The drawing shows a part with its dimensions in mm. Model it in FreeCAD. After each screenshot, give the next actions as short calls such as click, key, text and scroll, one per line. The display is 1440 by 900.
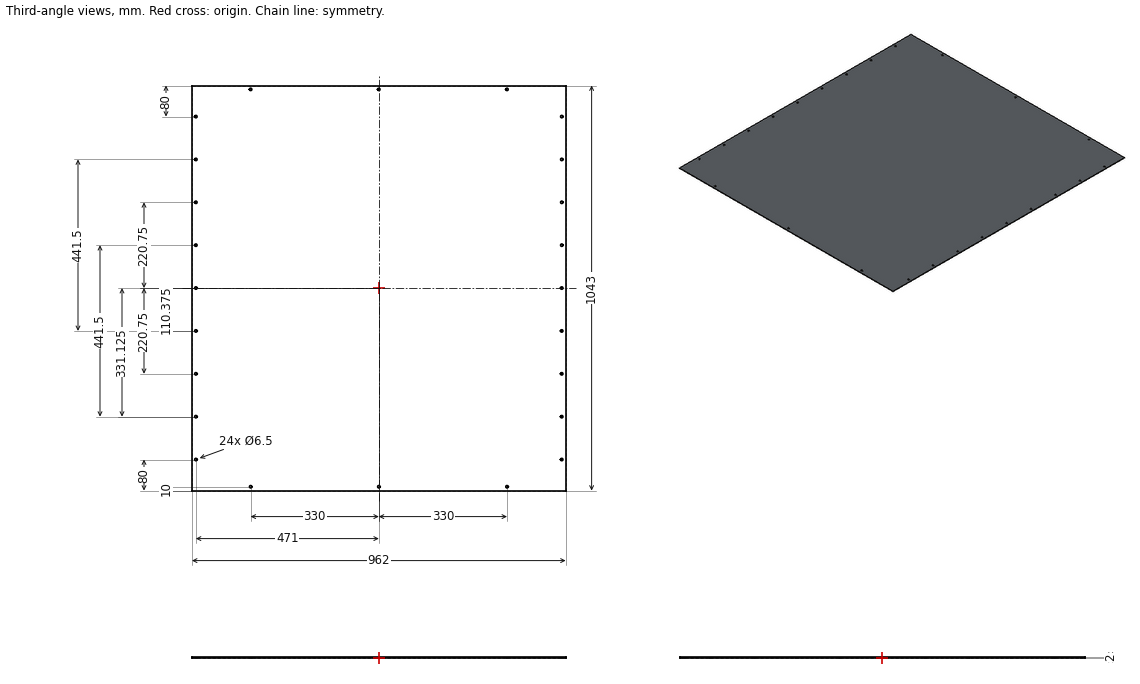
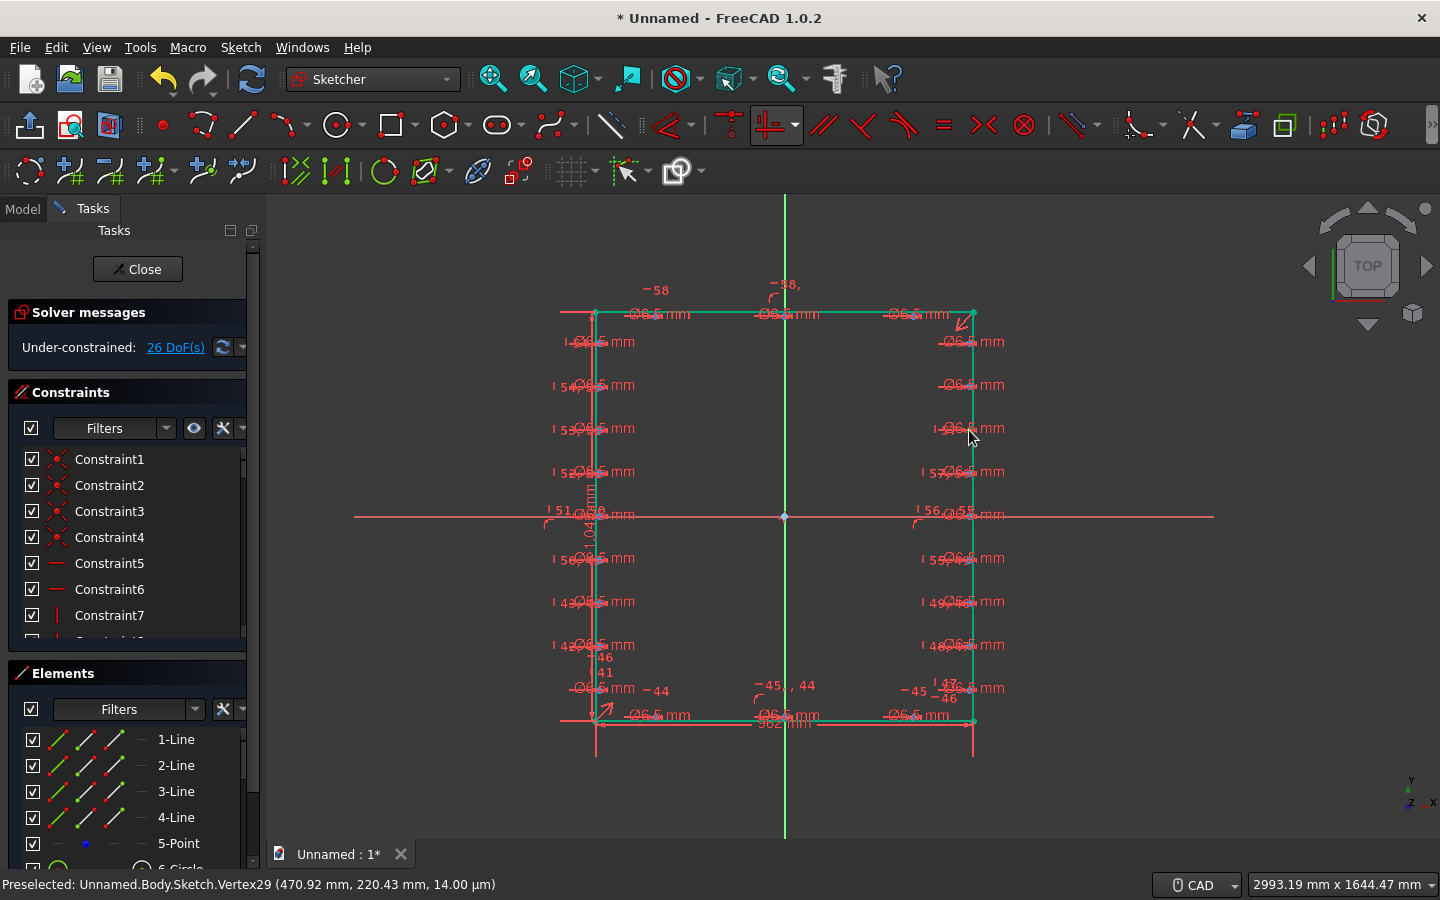
click(969, 387)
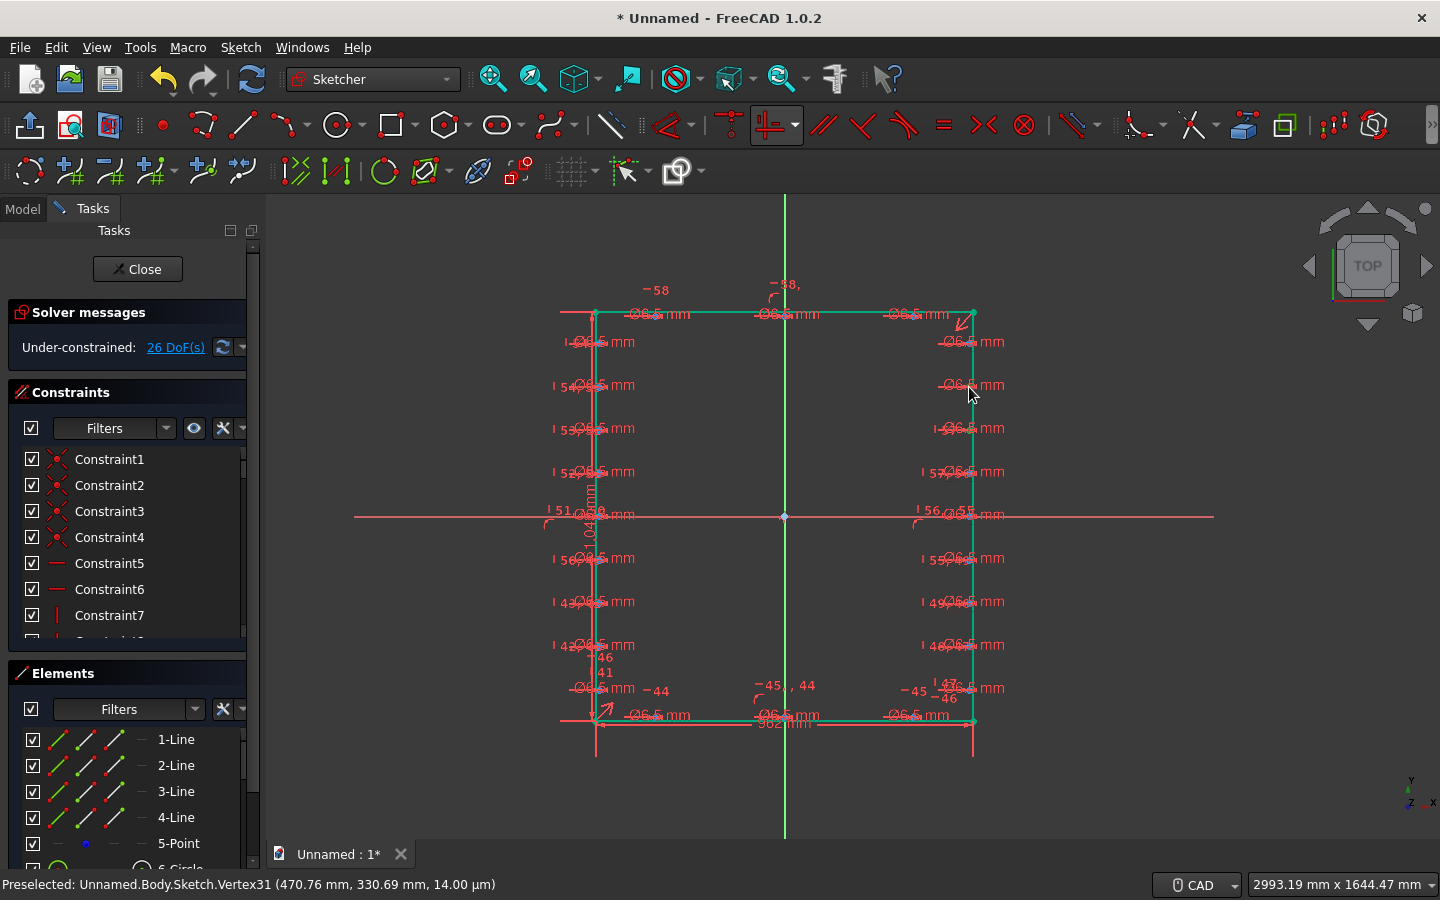
click(798, 126)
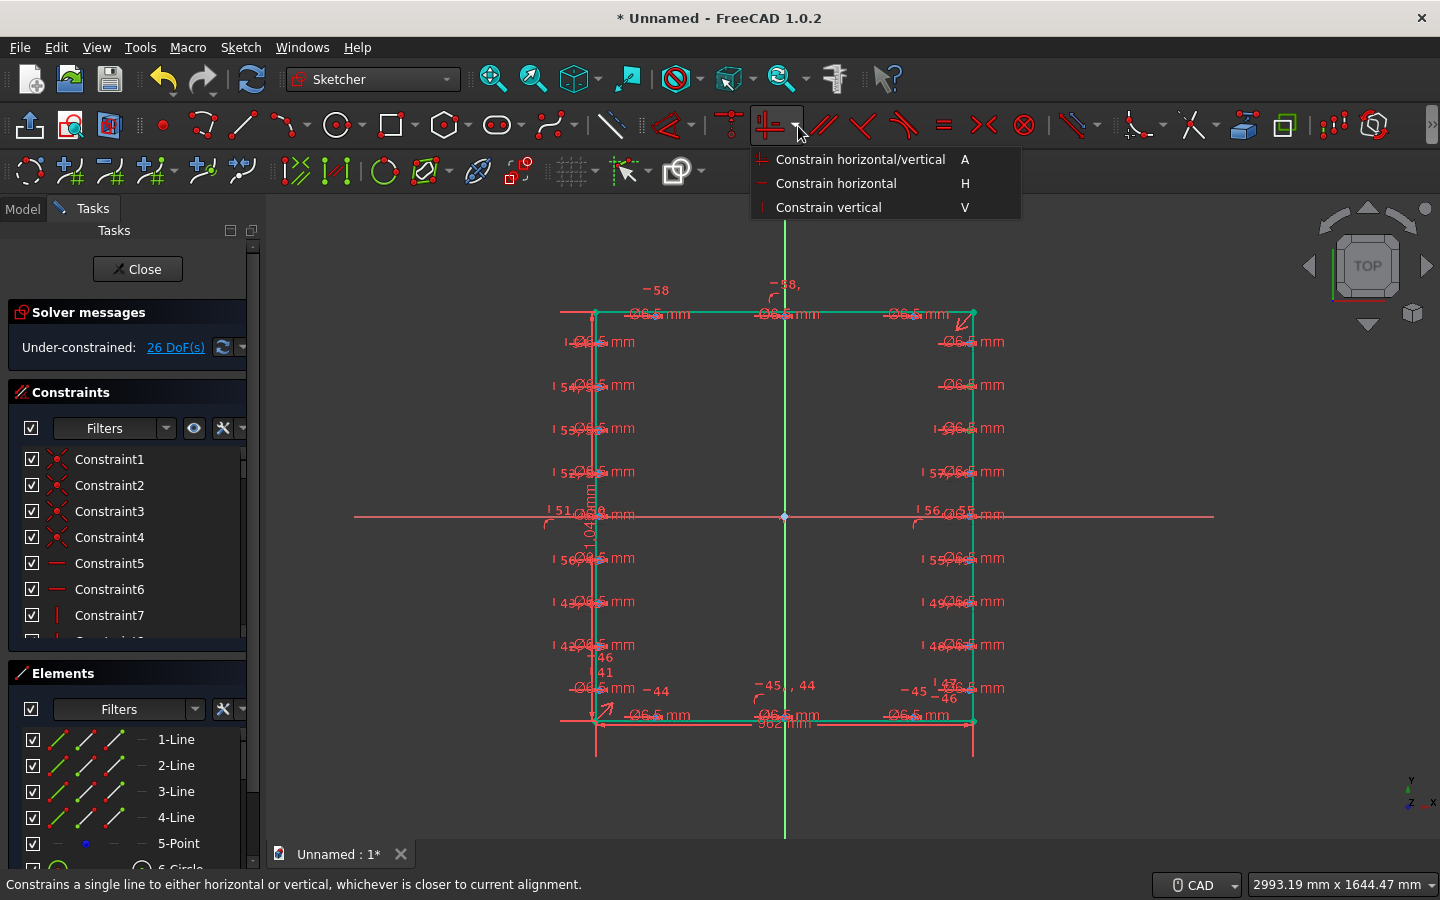
click(886, 207)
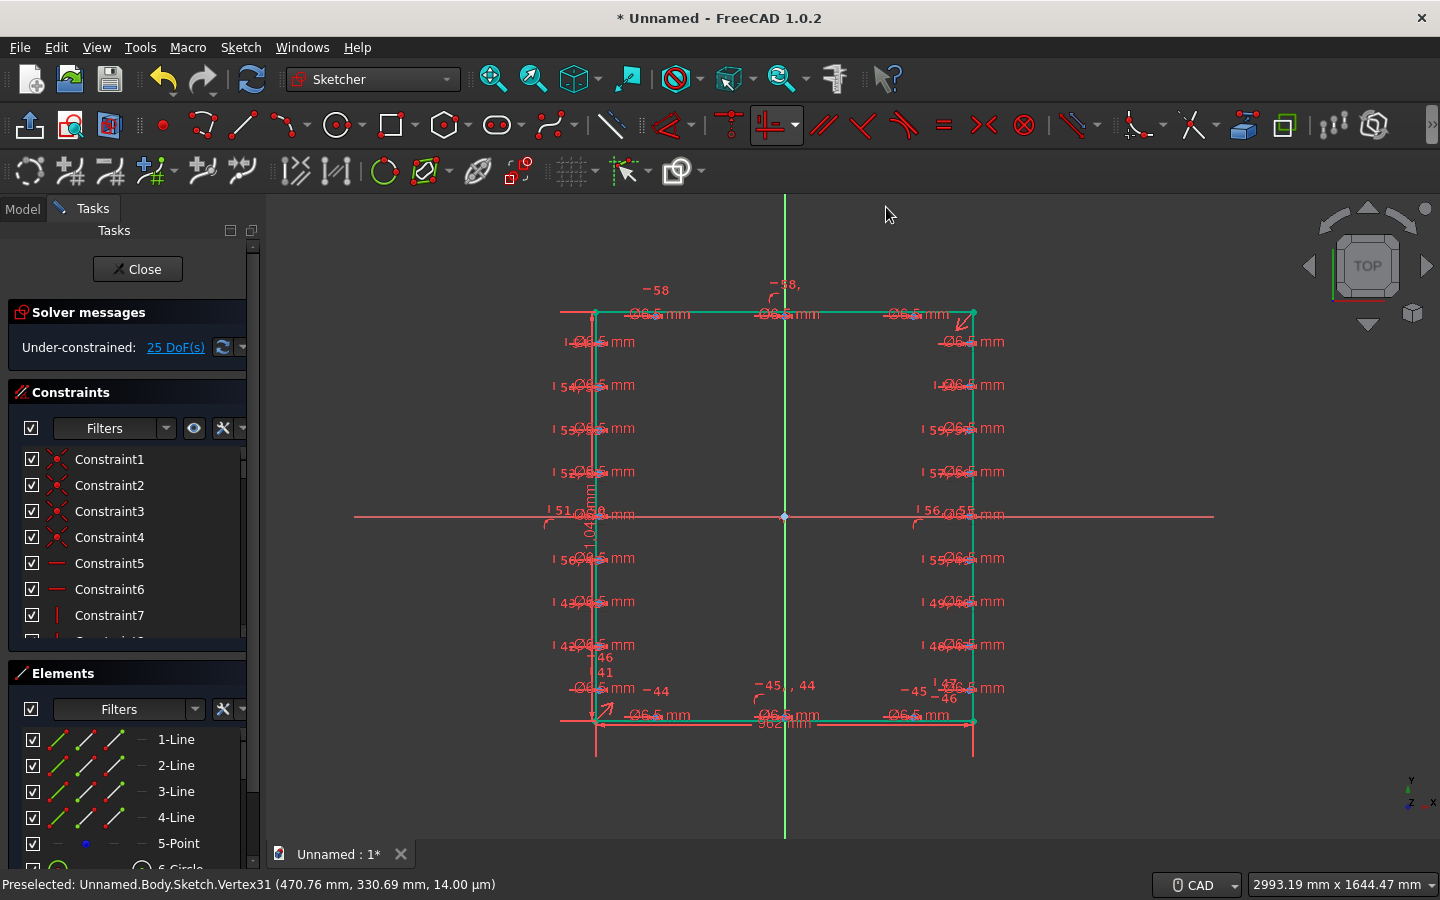
click(785, 316)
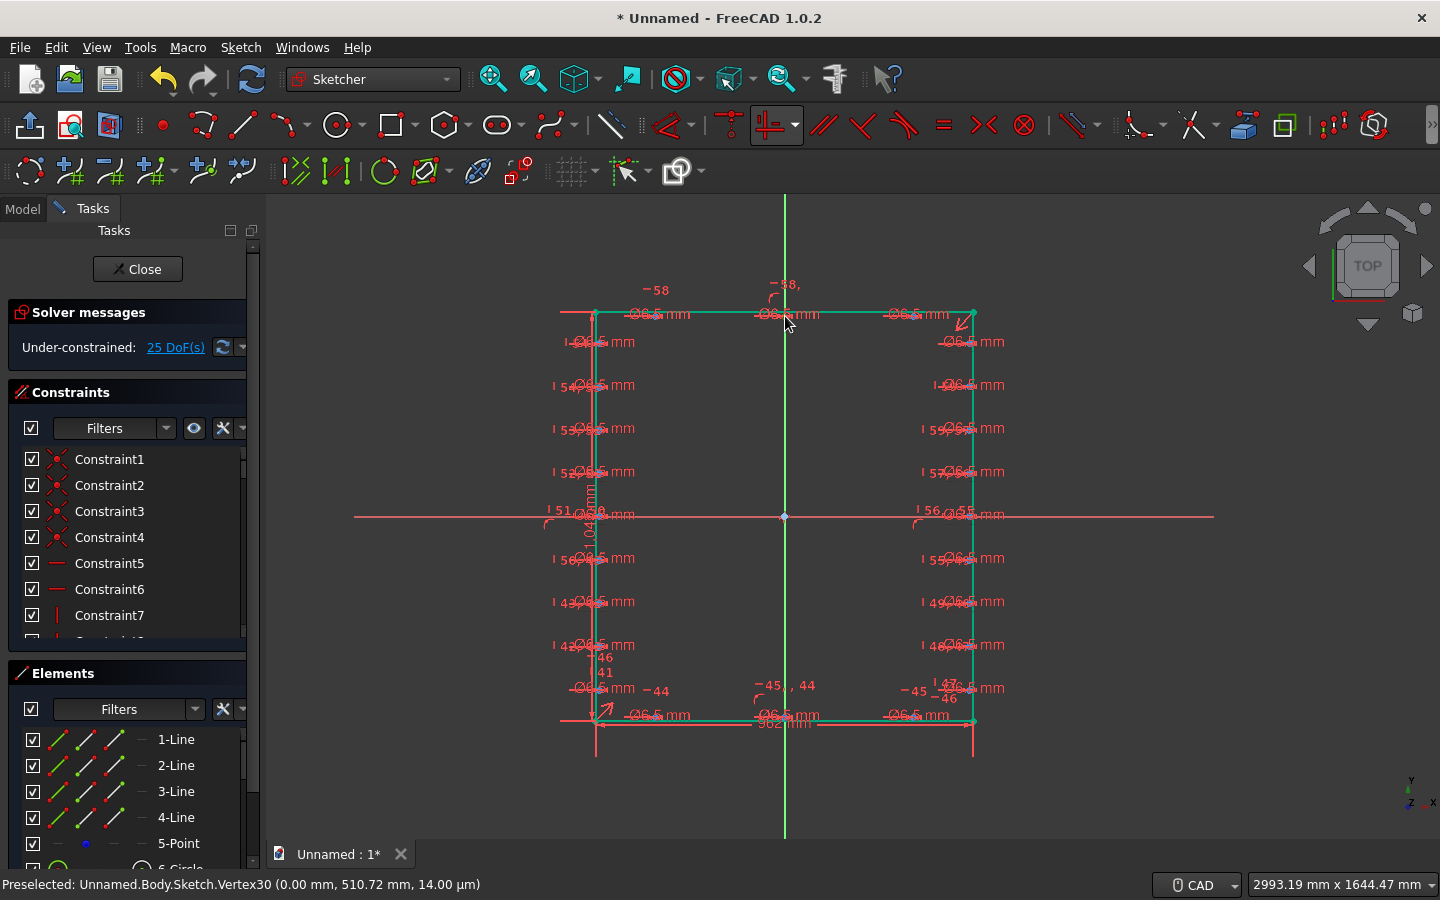
click(914, 316)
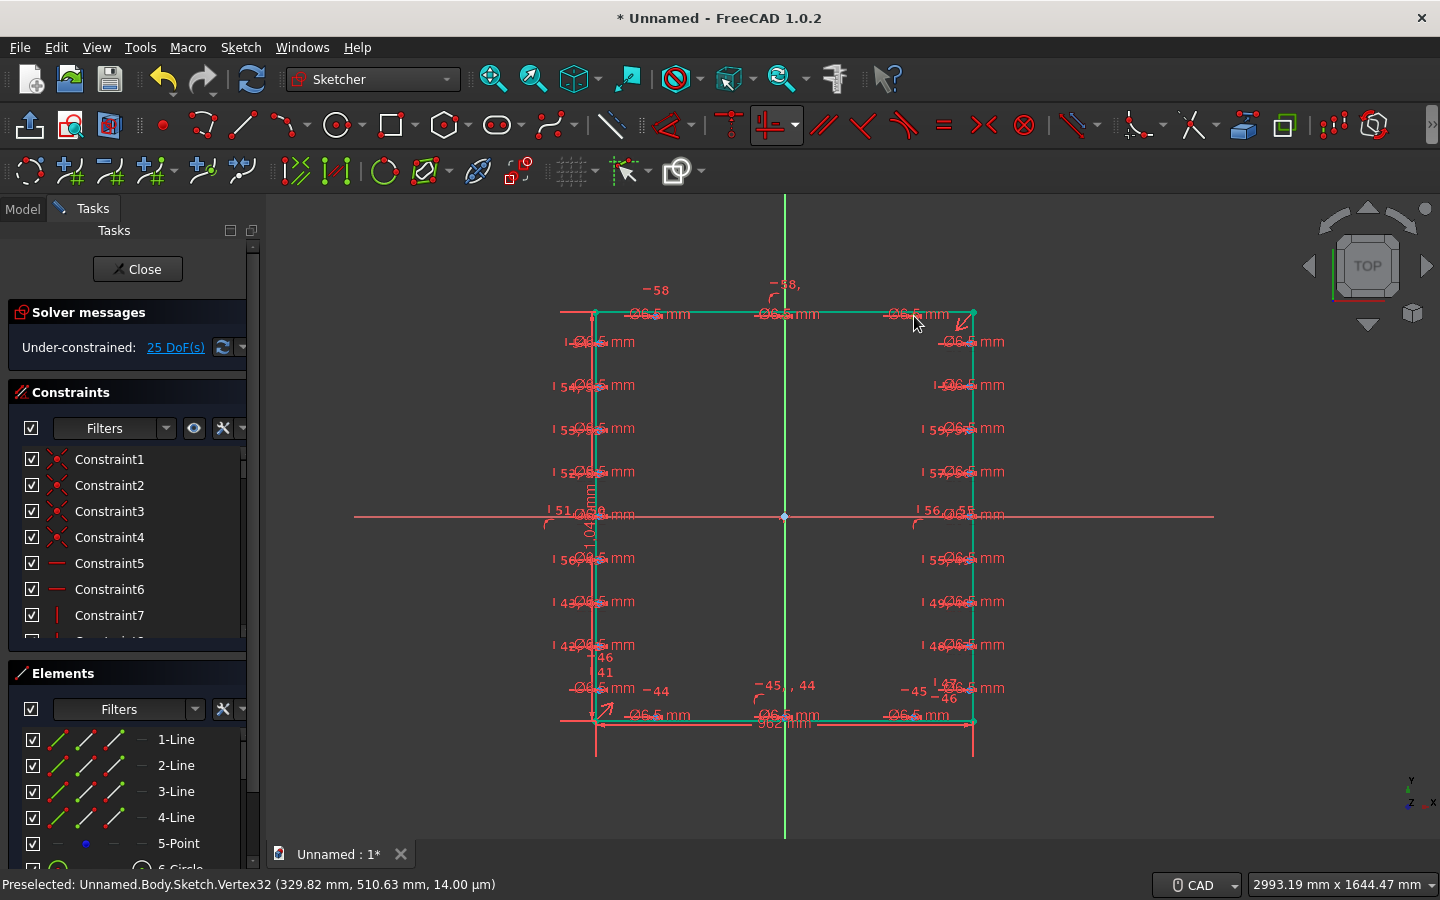
click(798, 126)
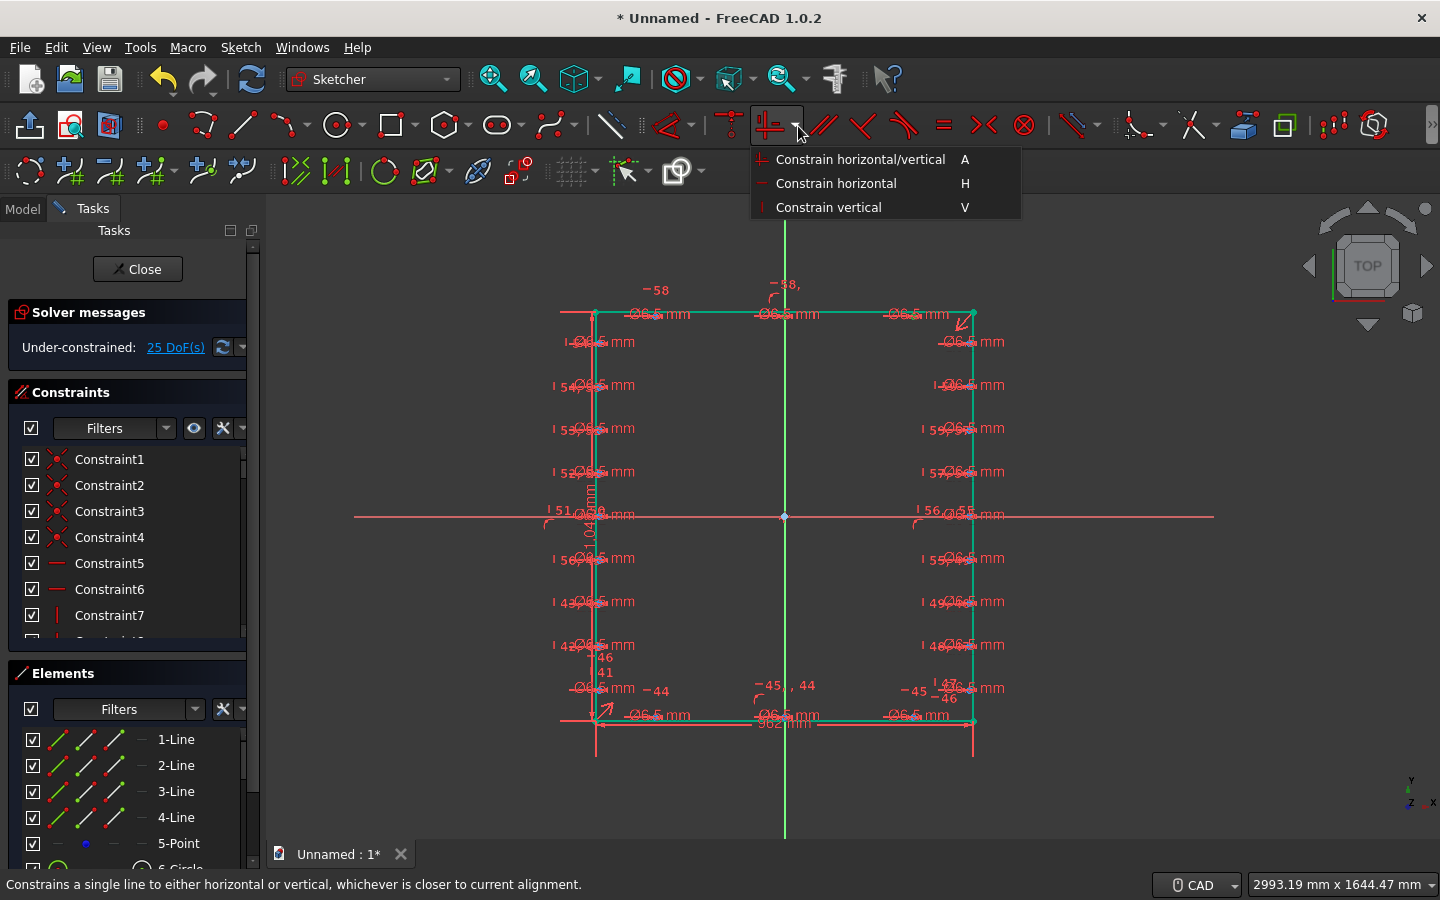
click(886, 183)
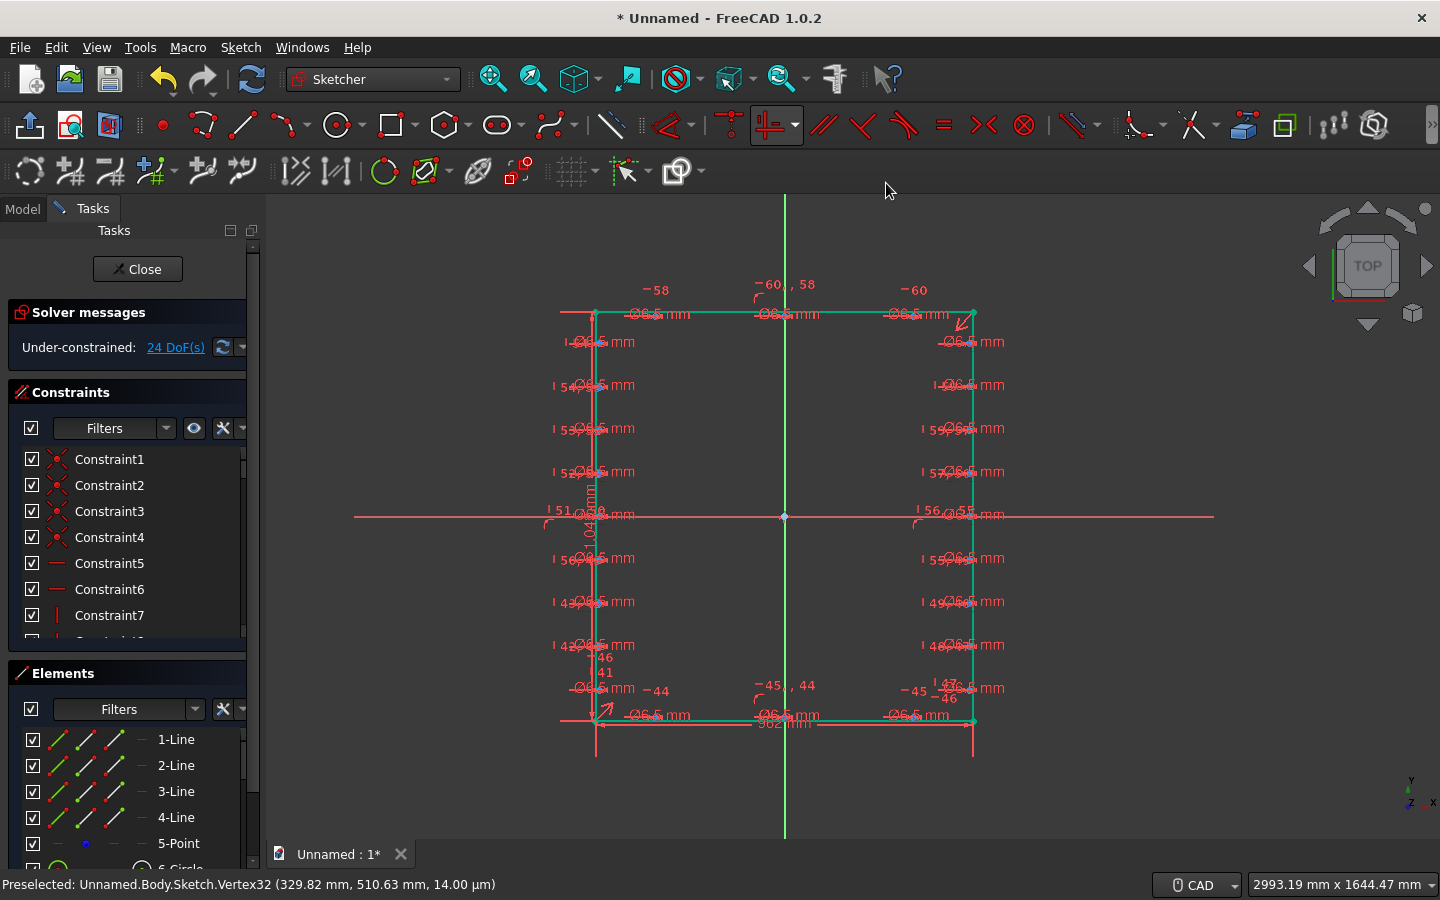
click(969, 387)